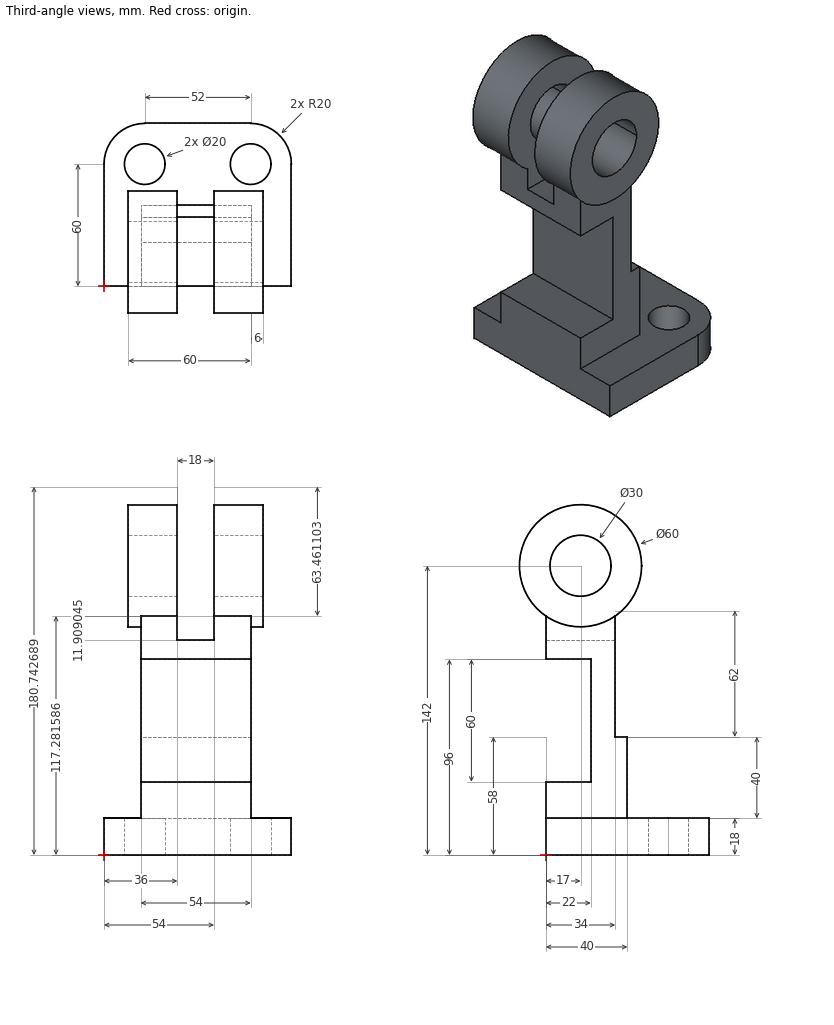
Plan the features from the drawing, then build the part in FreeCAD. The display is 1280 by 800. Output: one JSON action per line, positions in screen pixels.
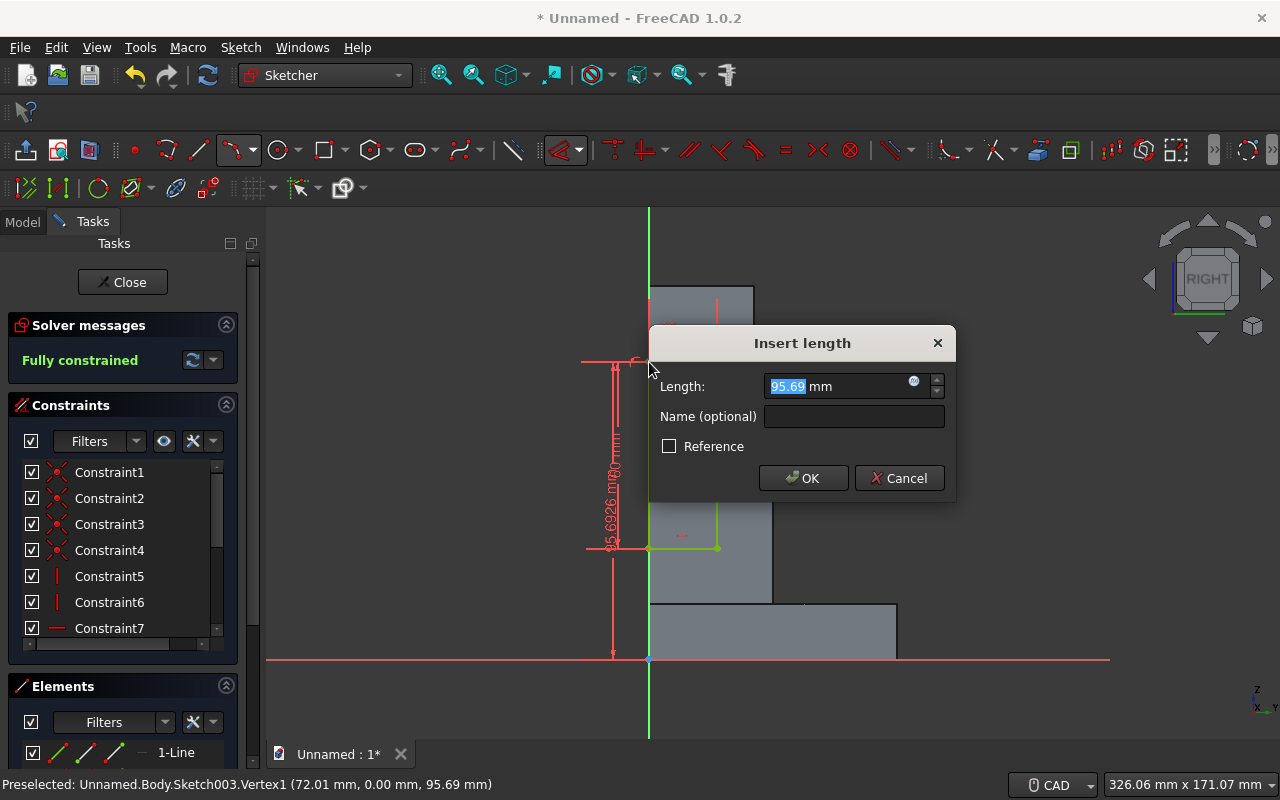
{"action": "type", "text": "96"}
{"action": "key", "text": "Return"}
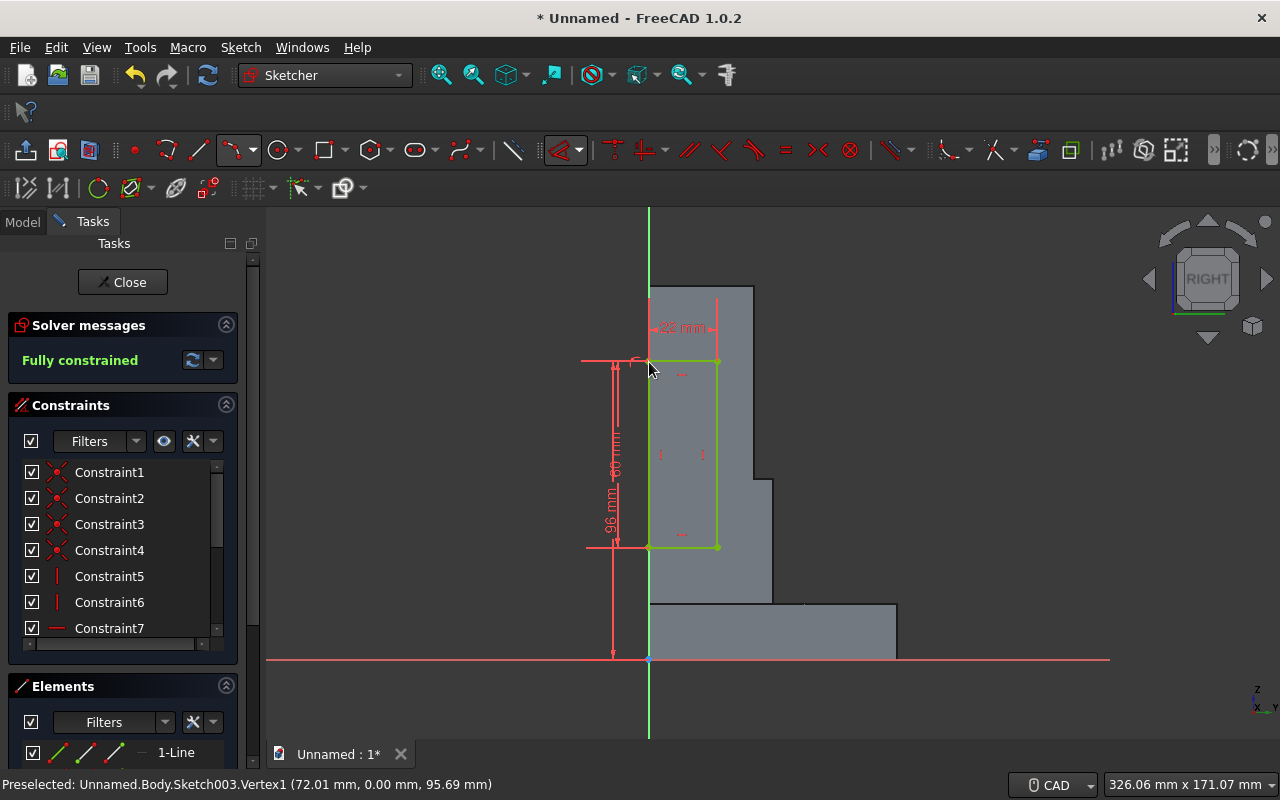
{"action": "left_click", "coordinate": [123, 282]}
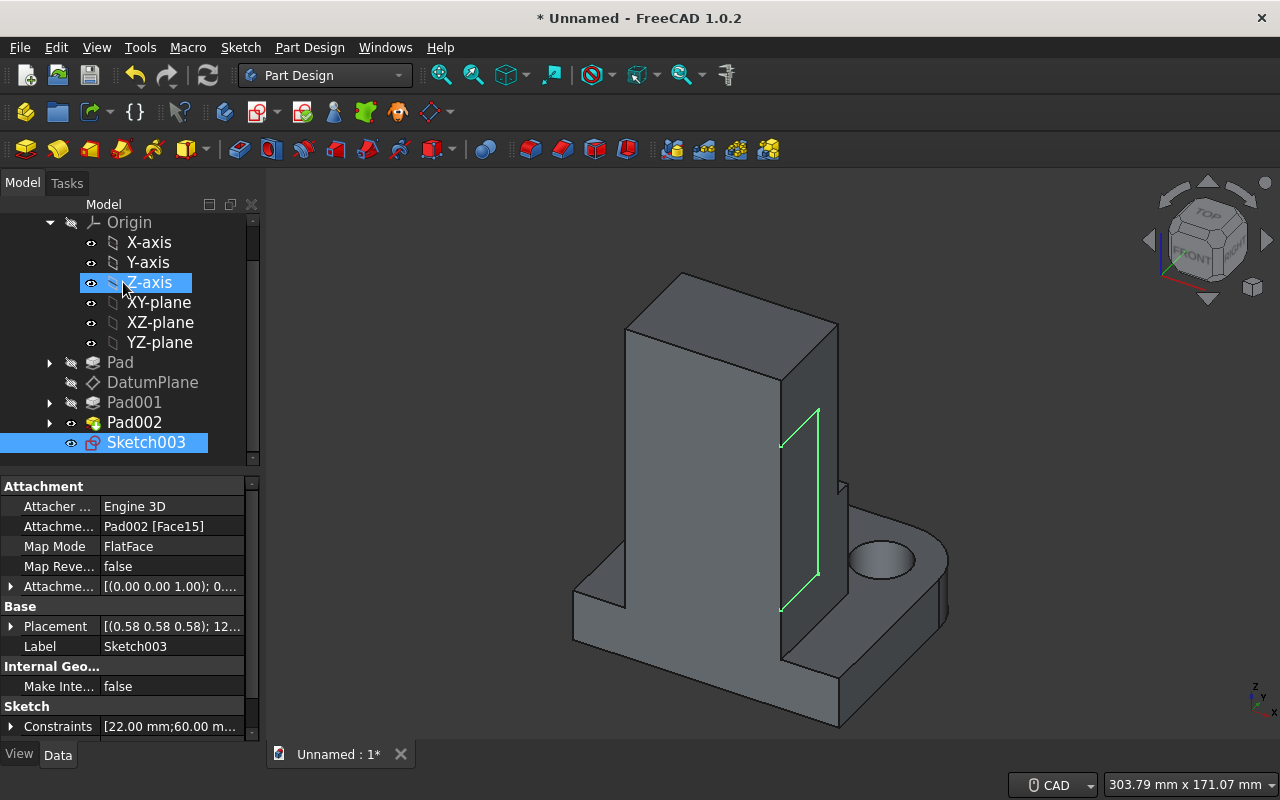
{"action": "left_click", "coordinate": [240, 150]}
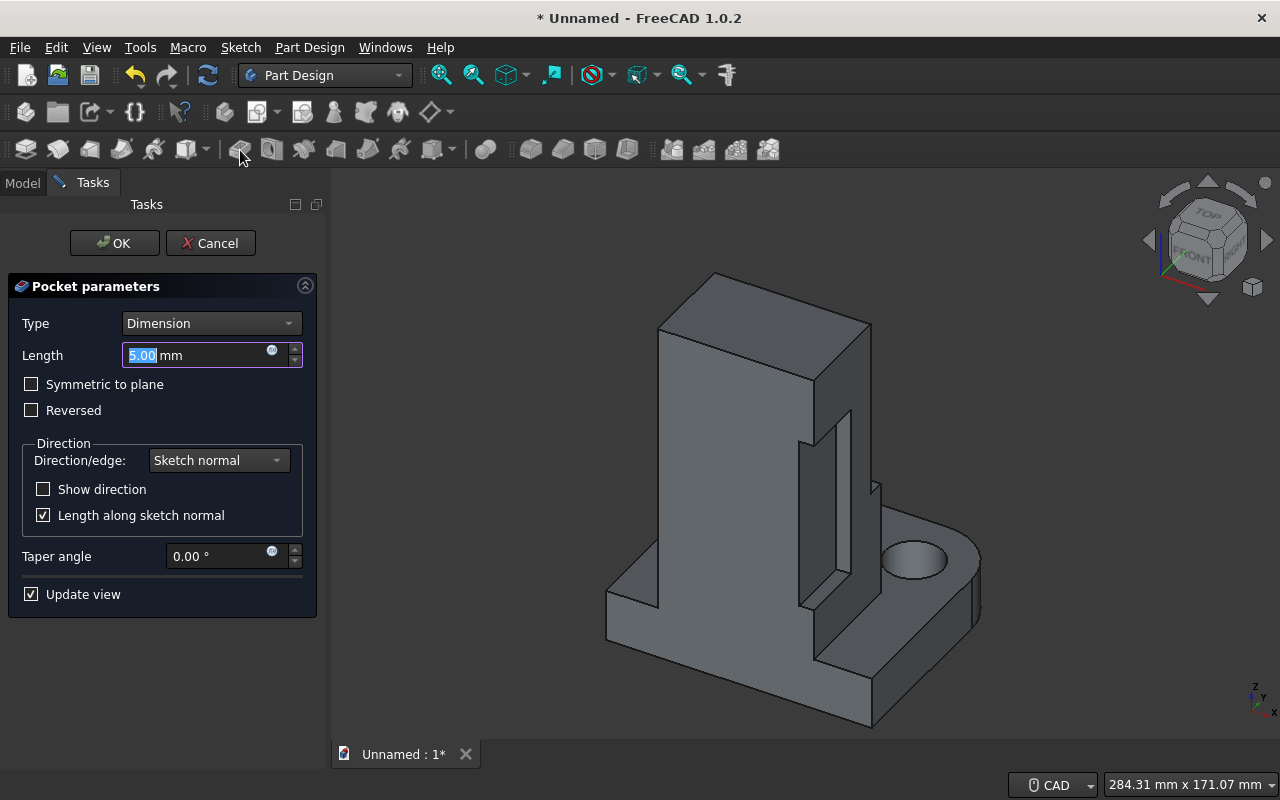
{"action": "type", "text": "54"}
{"action": "key", "text": "Tab"}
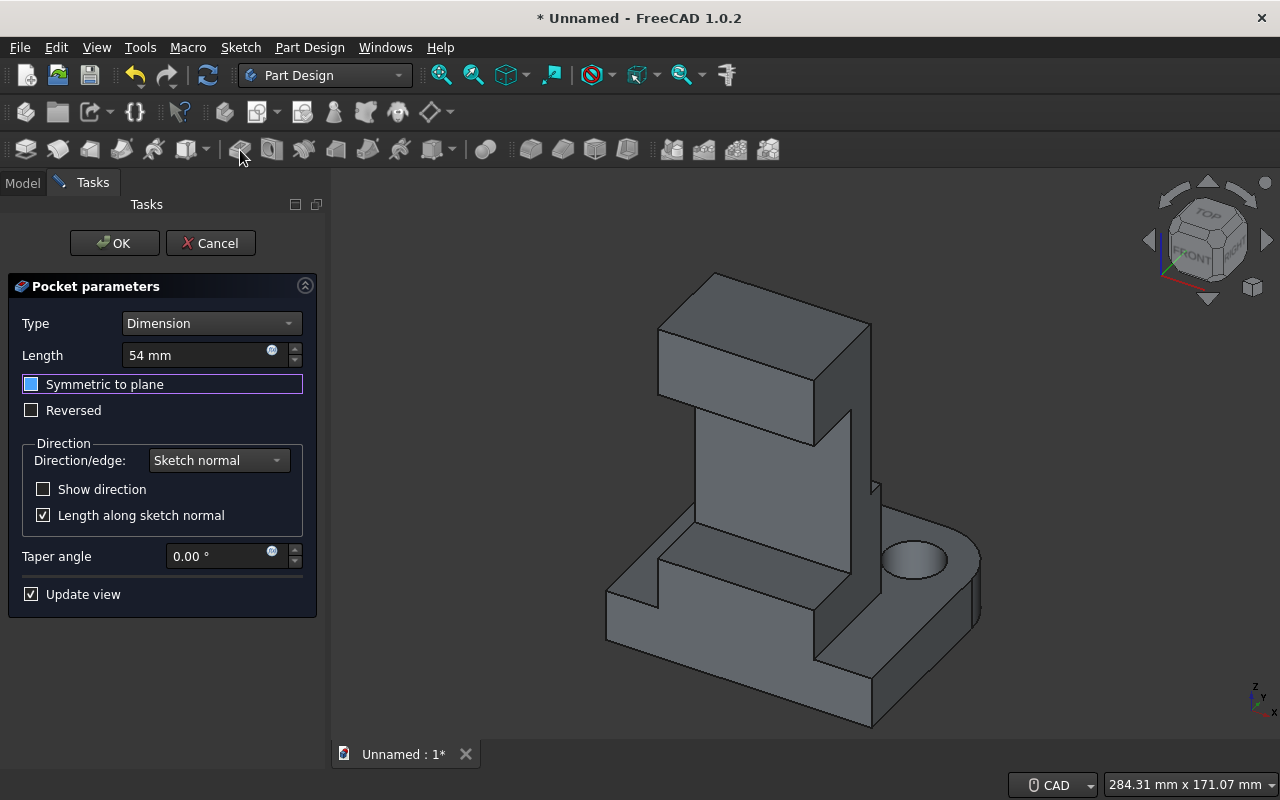
{"action": "left_click", "coordinate": [115, 243]}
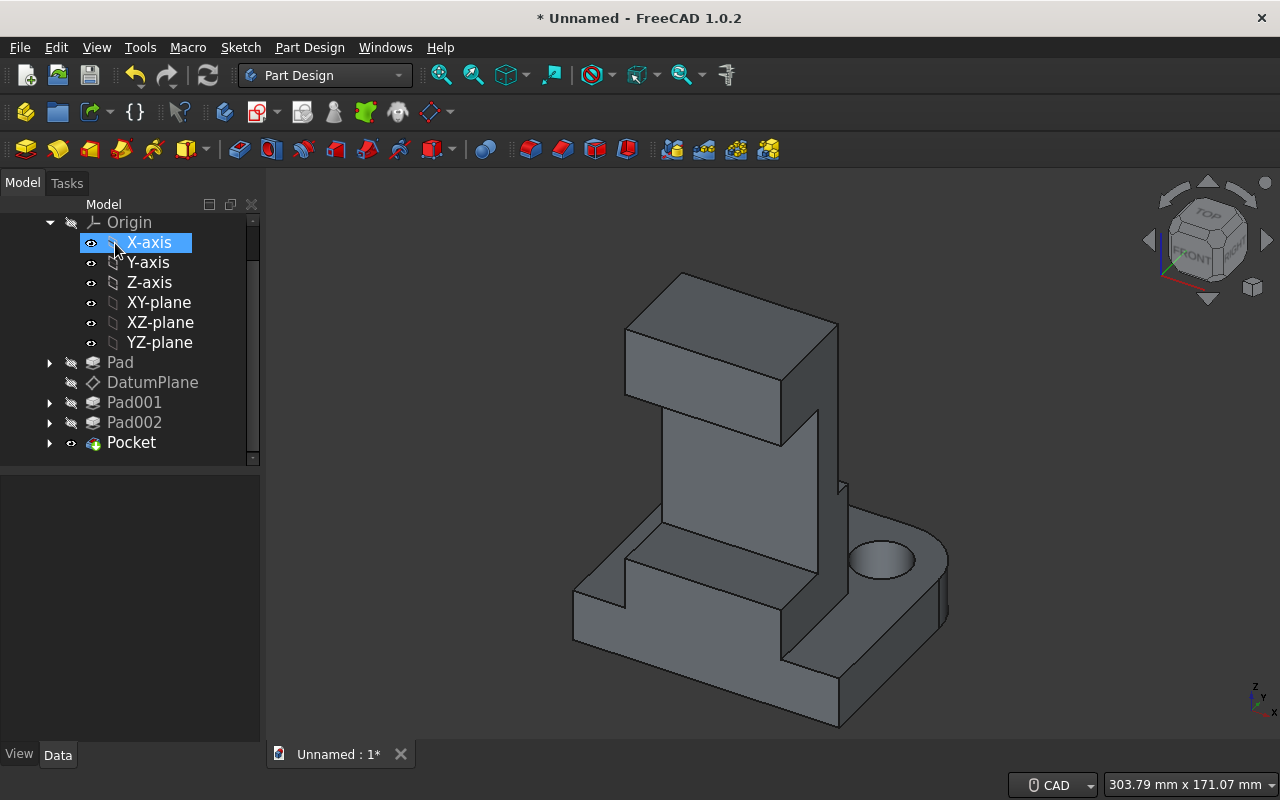
{"action": "left_click", "coordinate": [834, 547]}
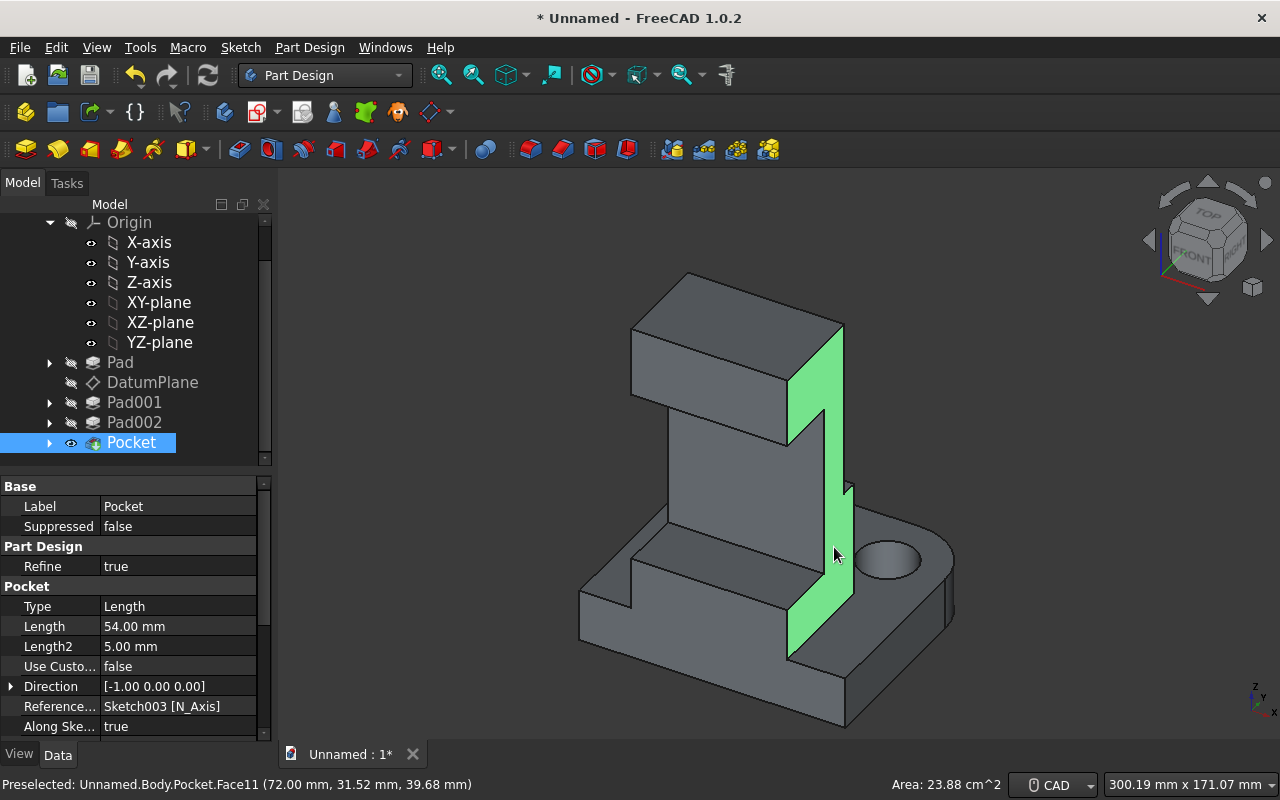
{"action": "left_click", "coordinate": [258, 112]}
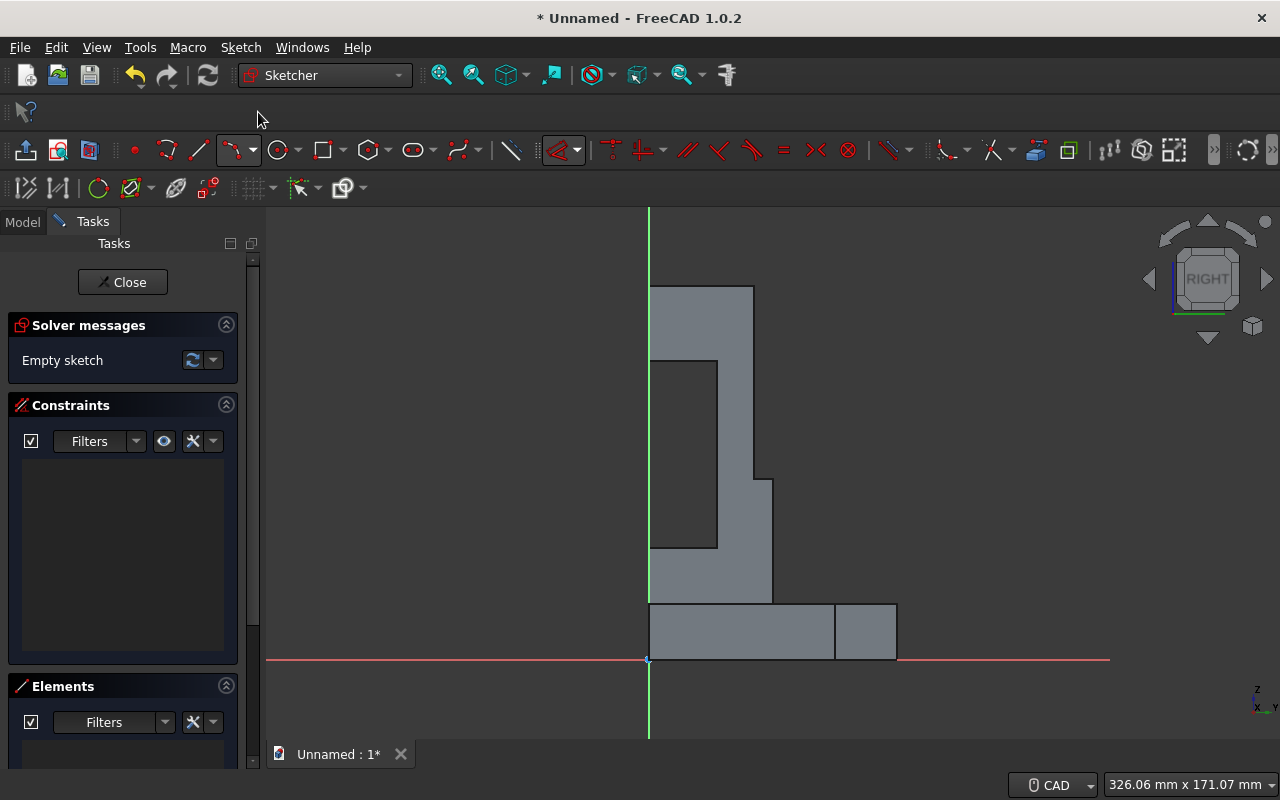
{"action": "left_click", "coordinate": [90, 150]}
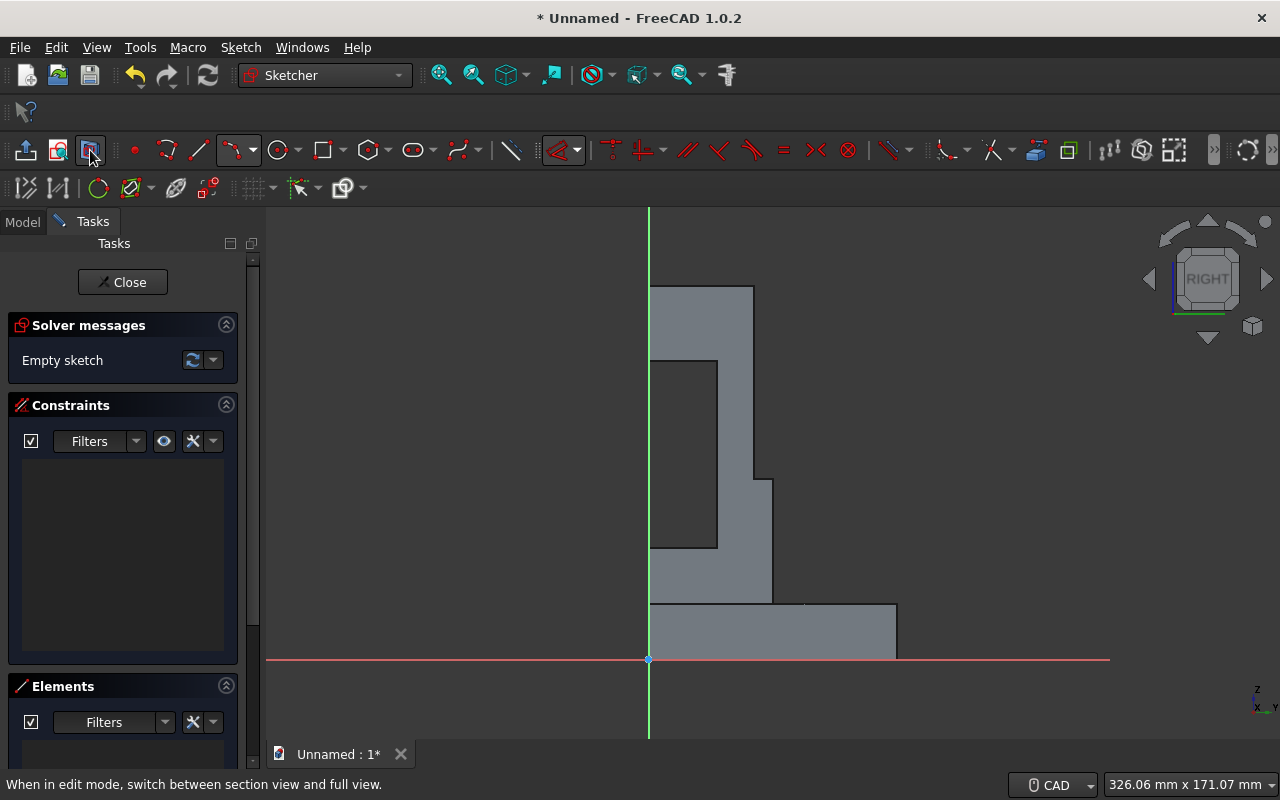
{"action": "scroll", "coordinate": [704, 473], "scroll_direction": "down", "scroll_amount": 5}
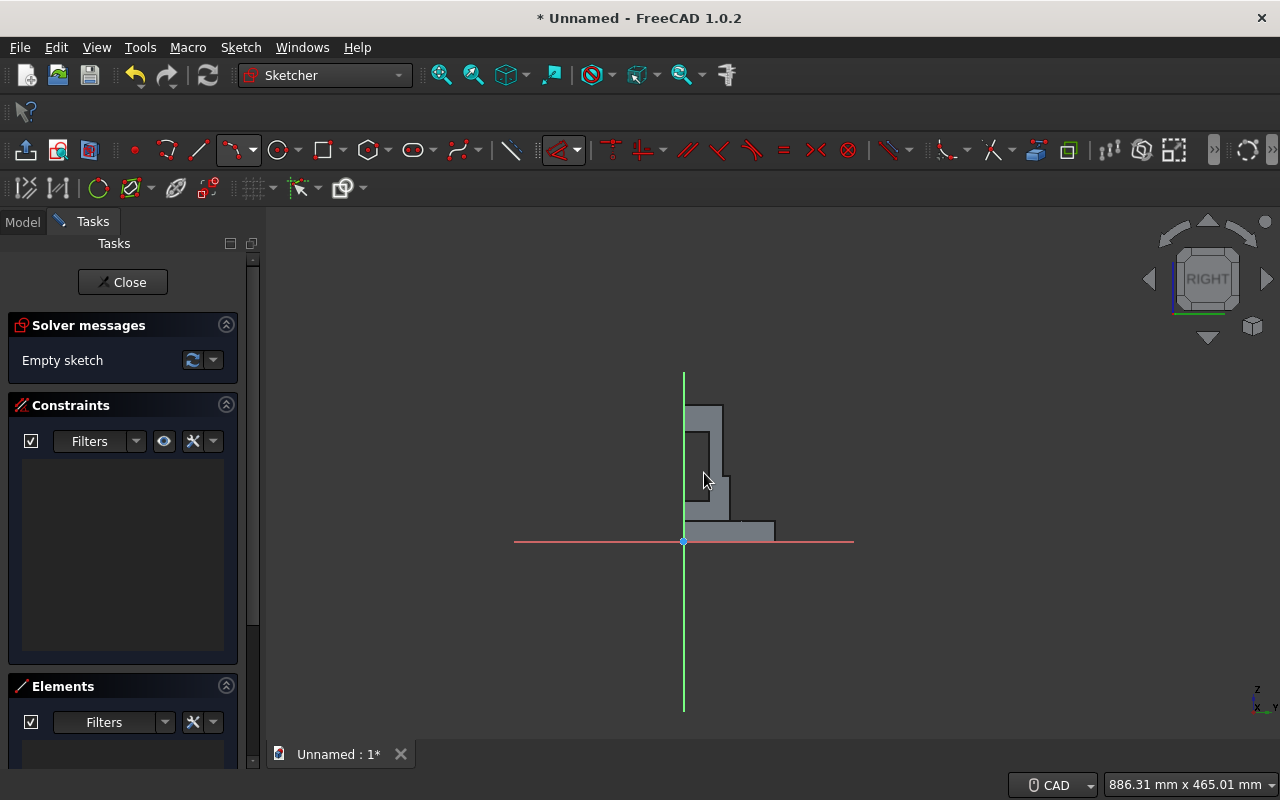
{"action": "scroll", "coordinate": [703, 356], "scroll_direction": "up", "scroll_amount": 8}